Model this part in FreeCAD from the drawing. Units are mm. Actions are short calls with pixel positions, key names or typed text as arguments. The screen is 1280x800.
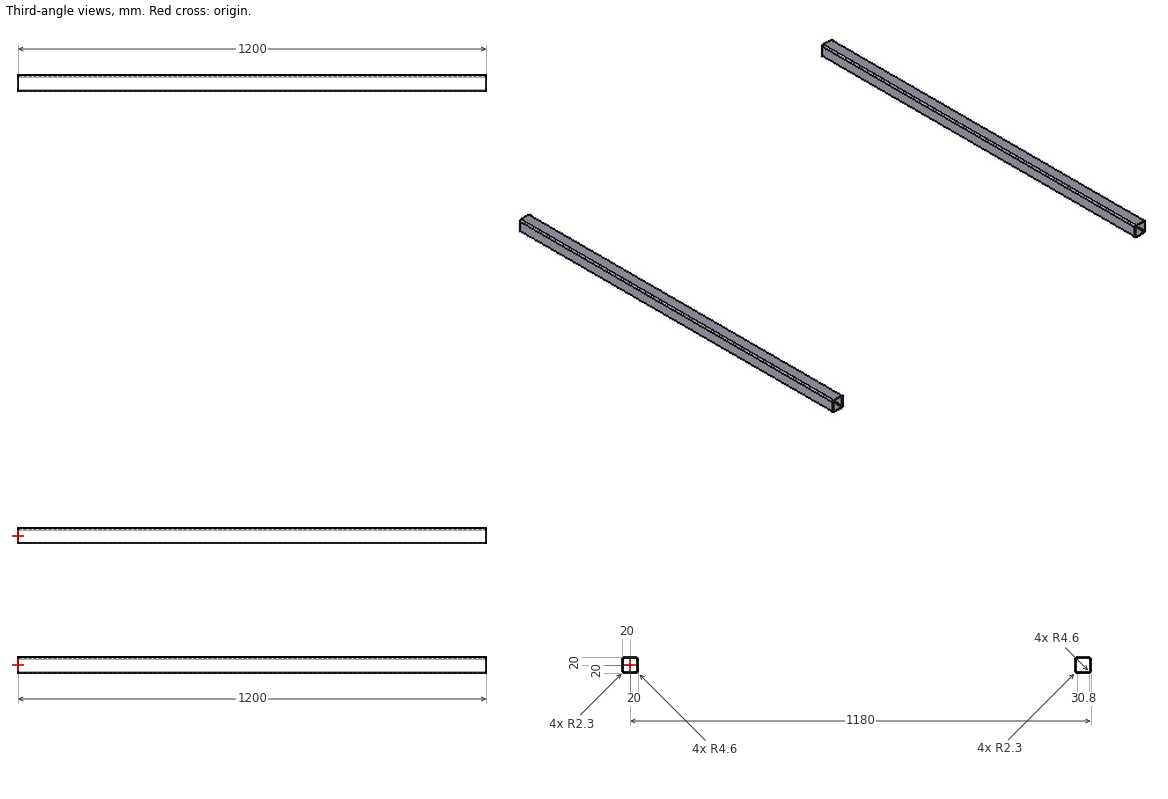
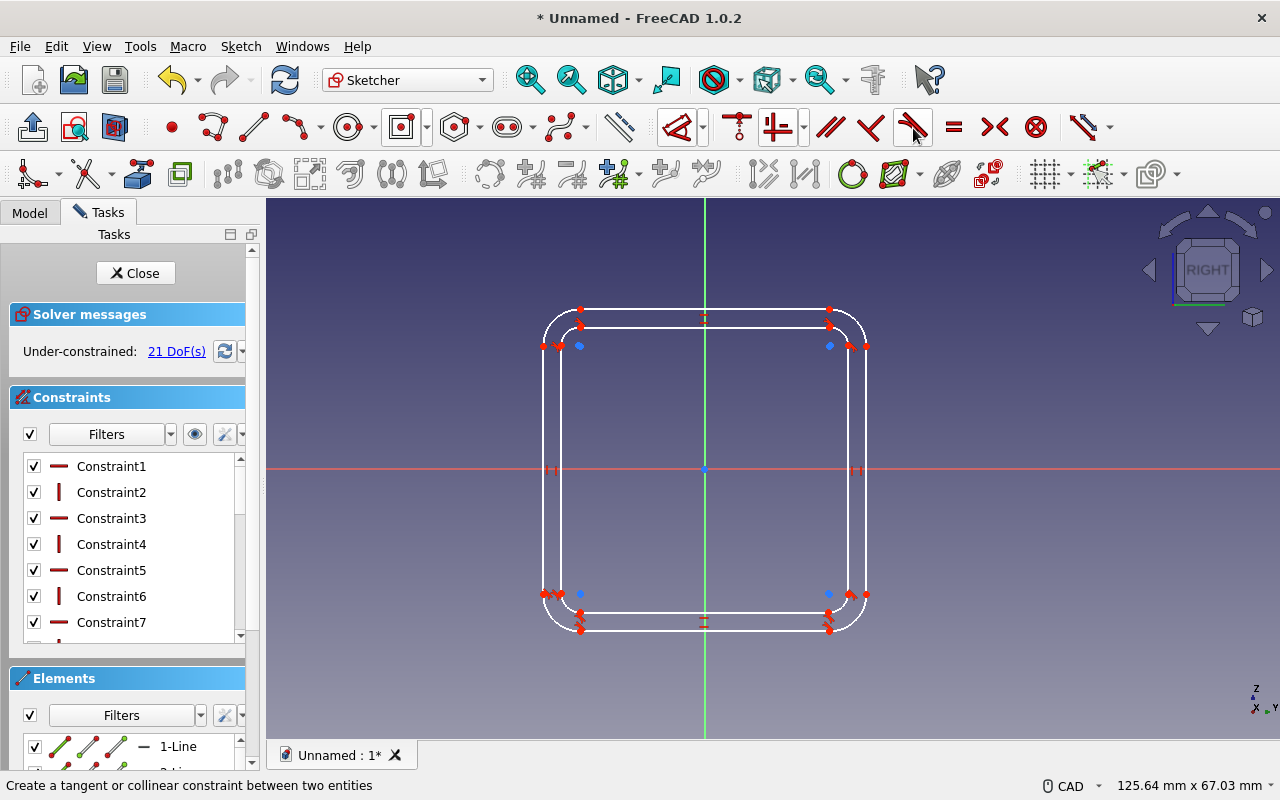
click(561, 519)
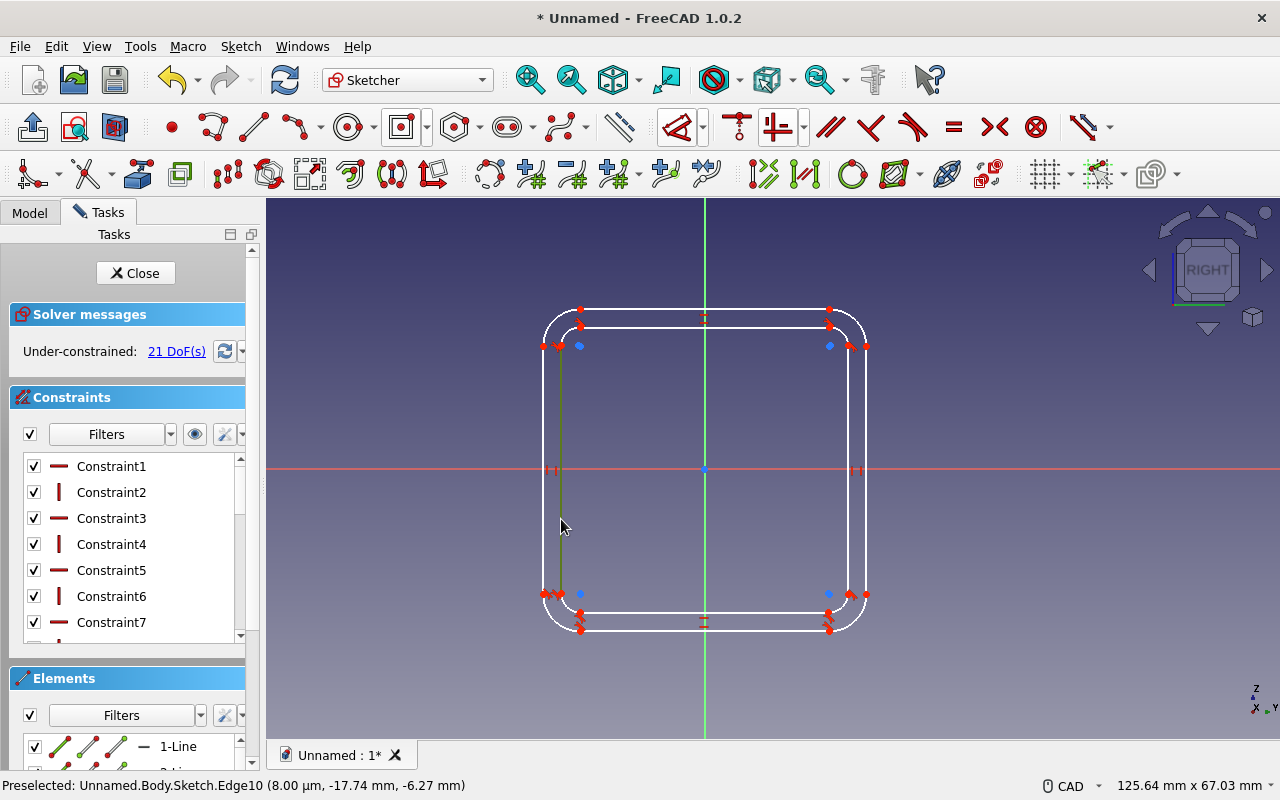
click(567, 333)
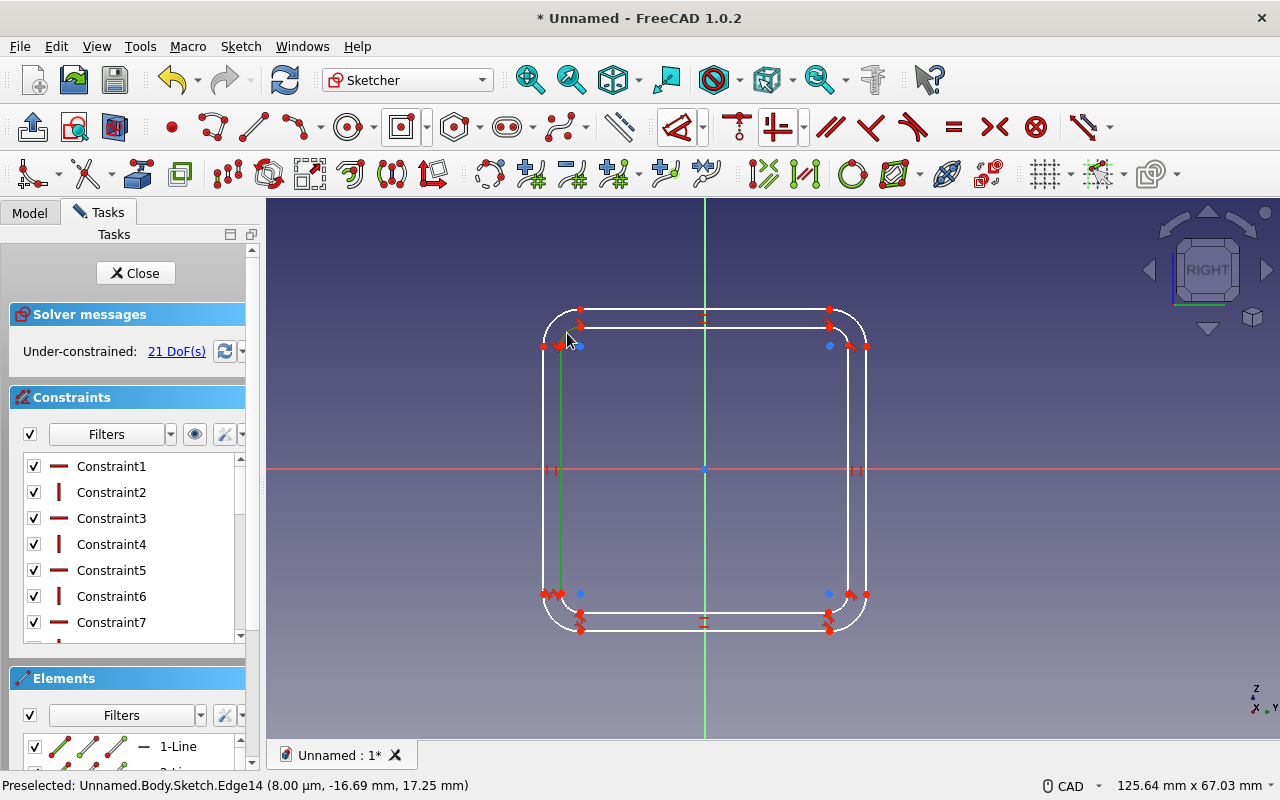
click(913, 128)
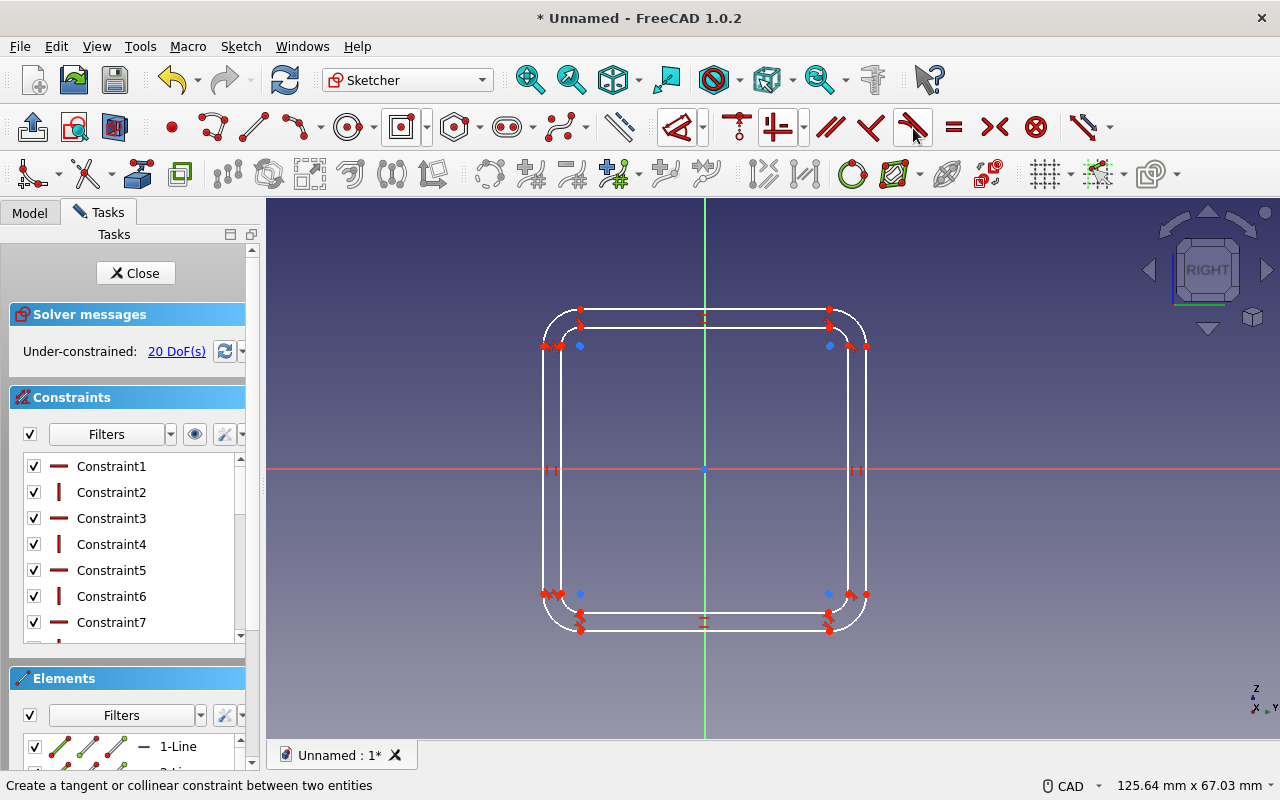
click(655, 328)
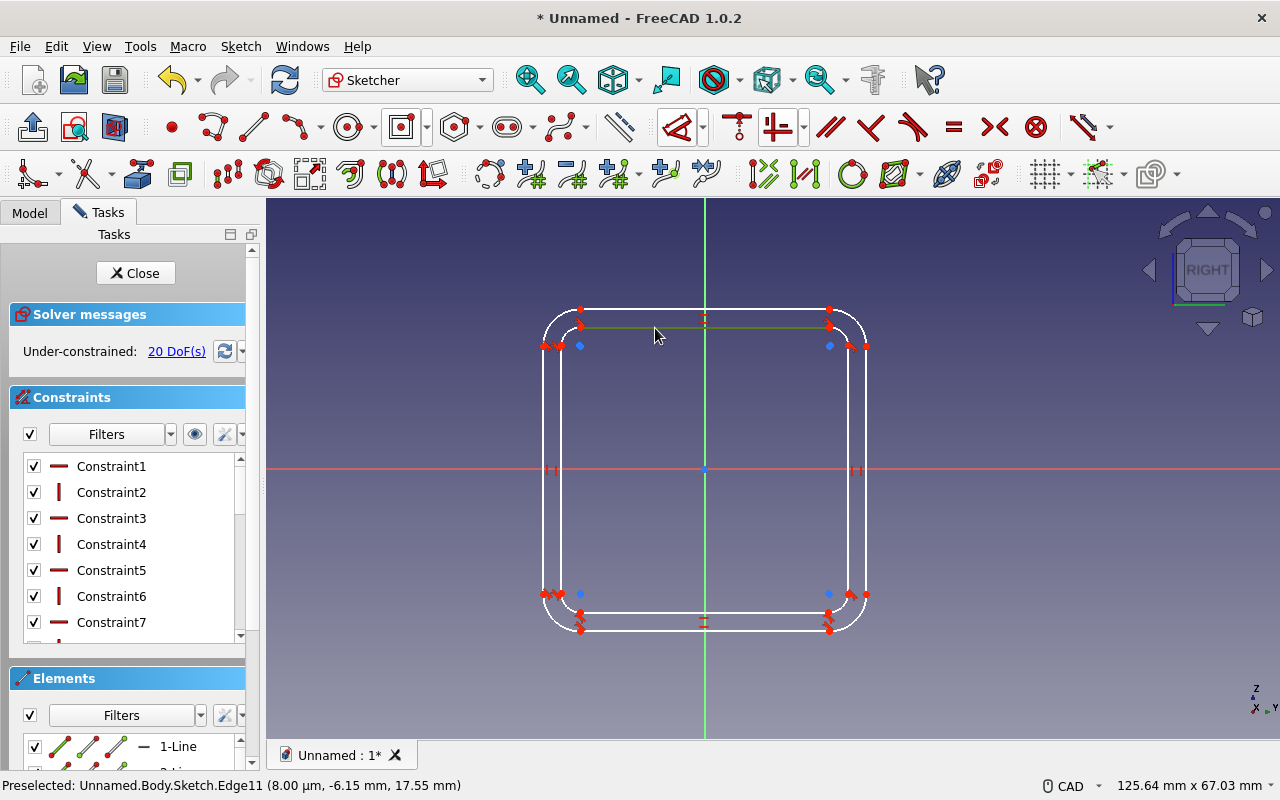
click(567, 333)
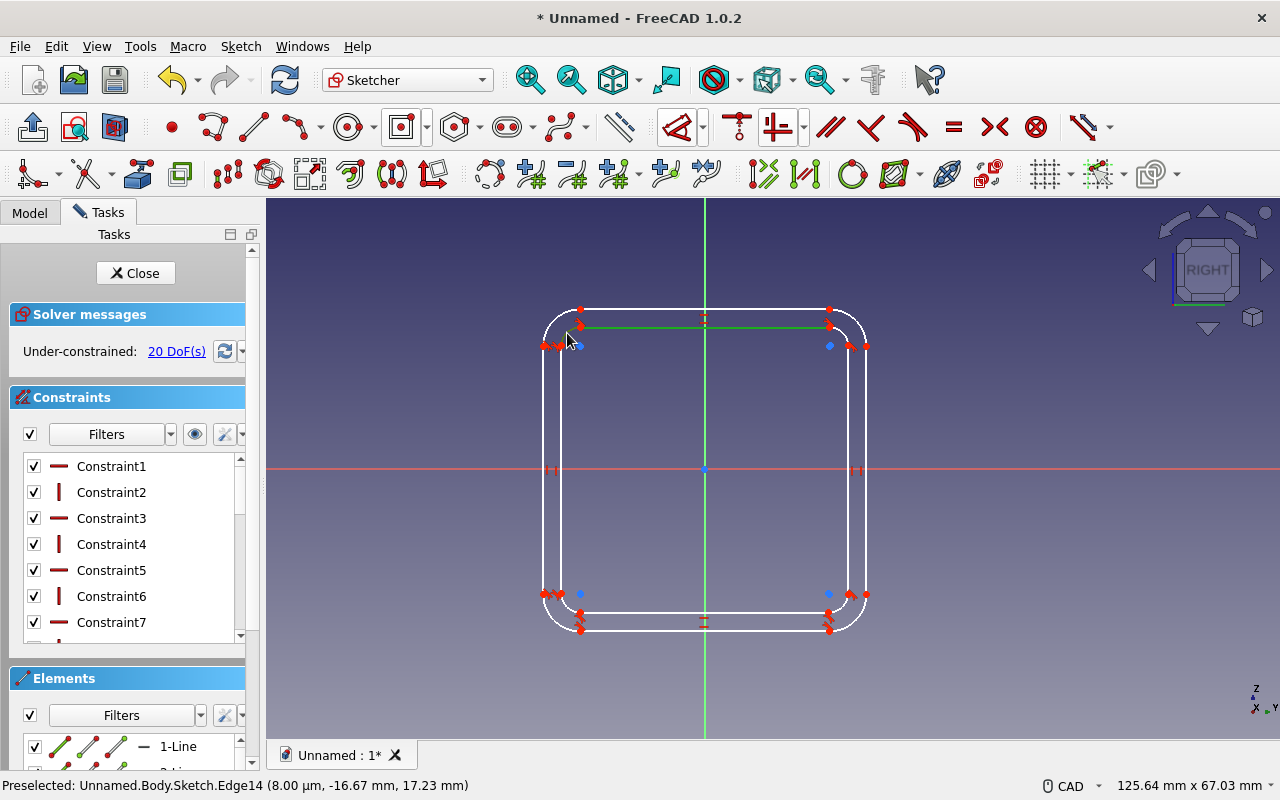
key(t)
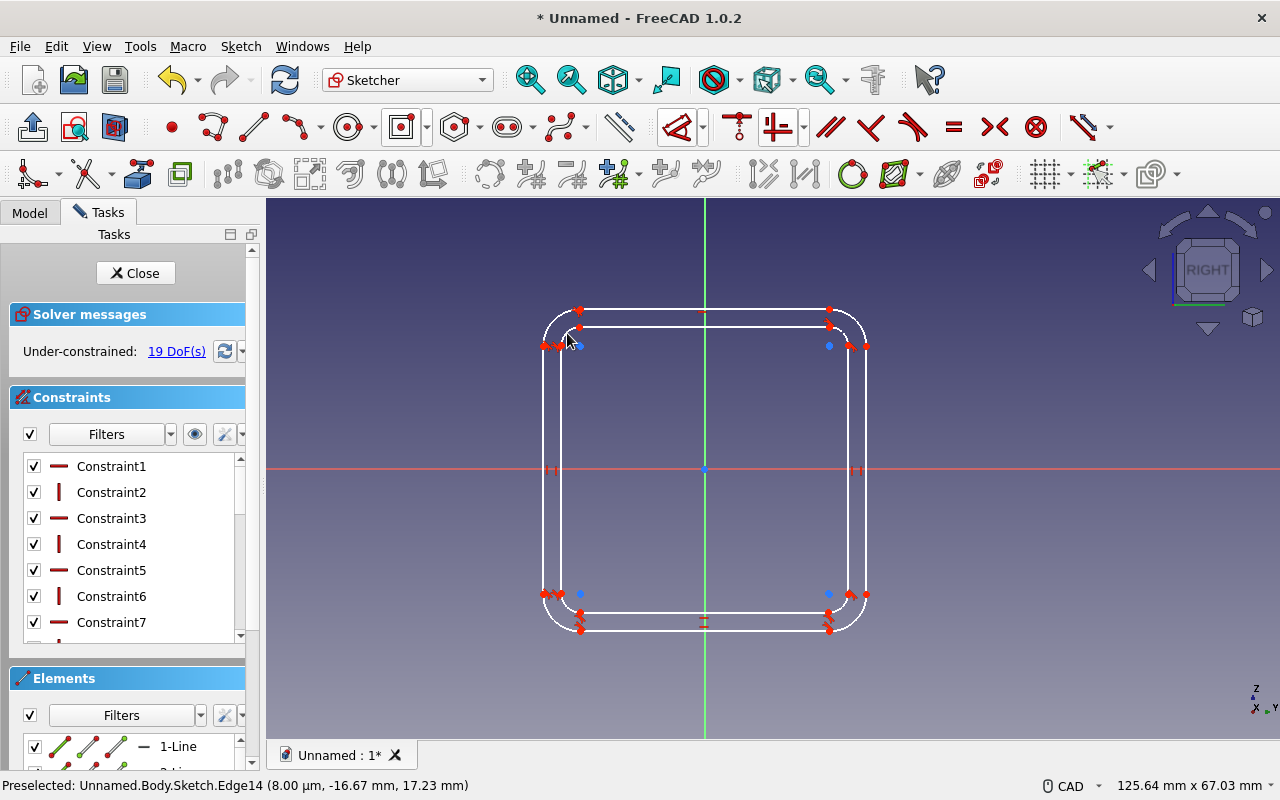
click(655, 327)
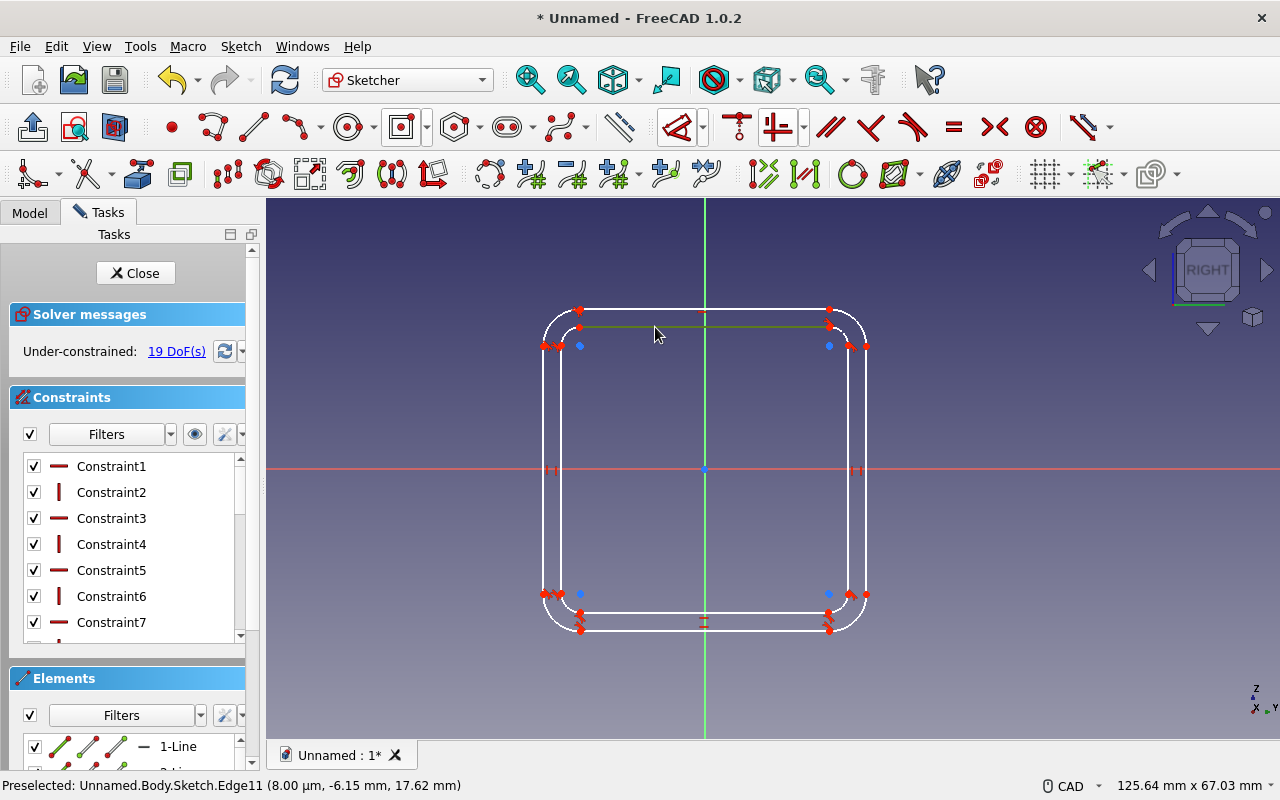
click(843, 332)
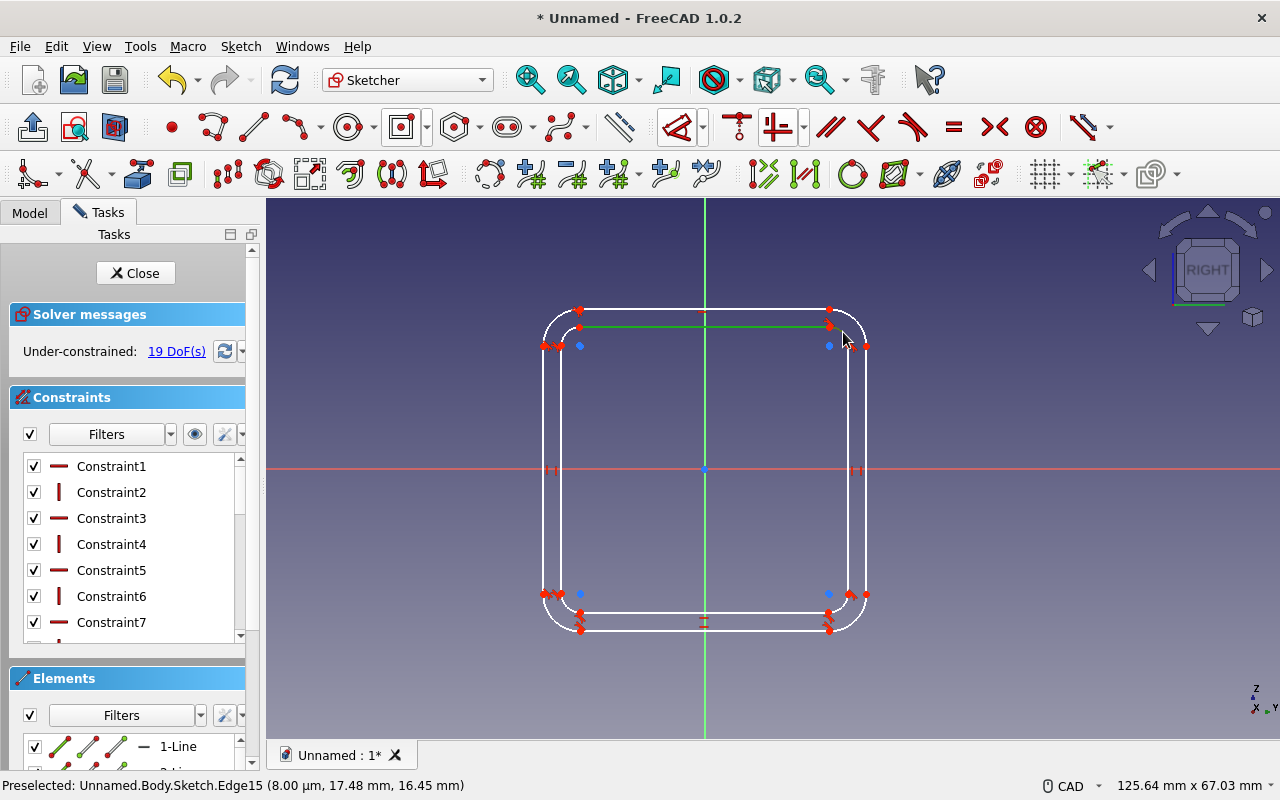
click(913, 128)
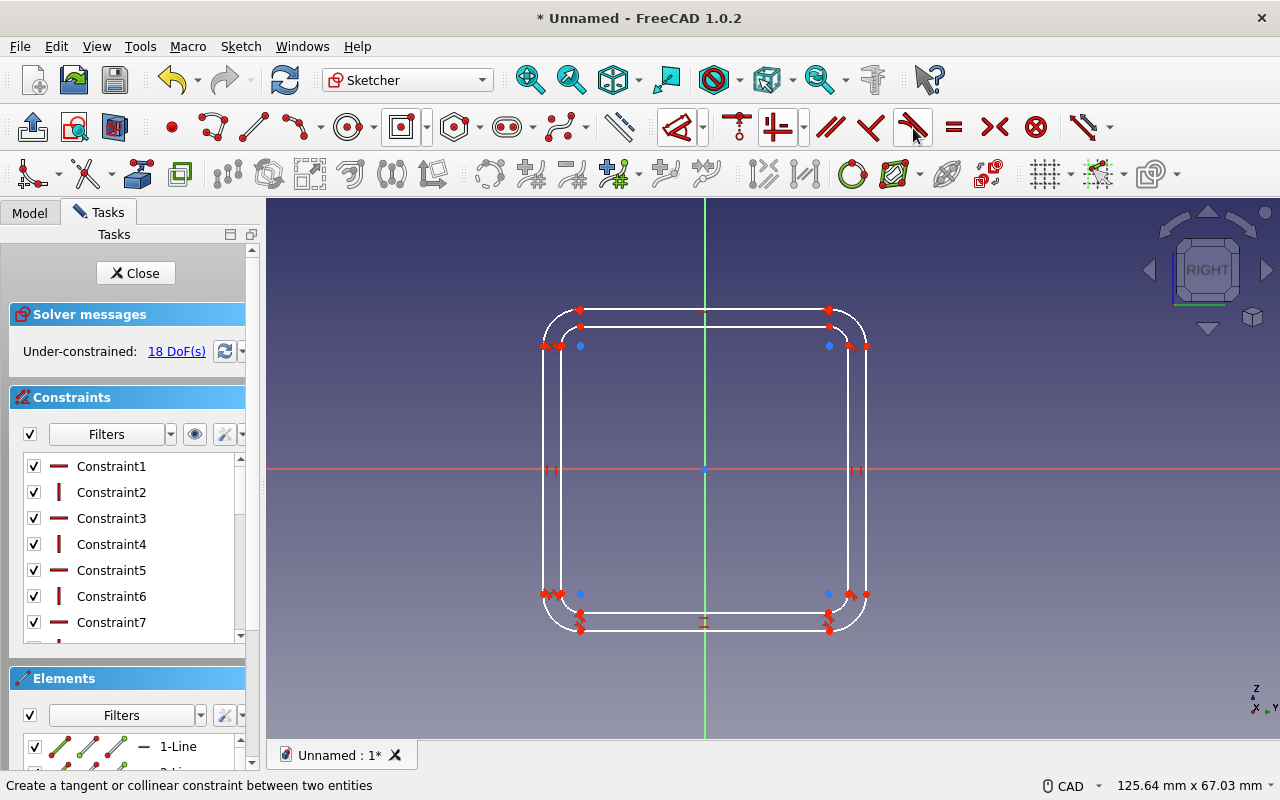
click(848, 420)